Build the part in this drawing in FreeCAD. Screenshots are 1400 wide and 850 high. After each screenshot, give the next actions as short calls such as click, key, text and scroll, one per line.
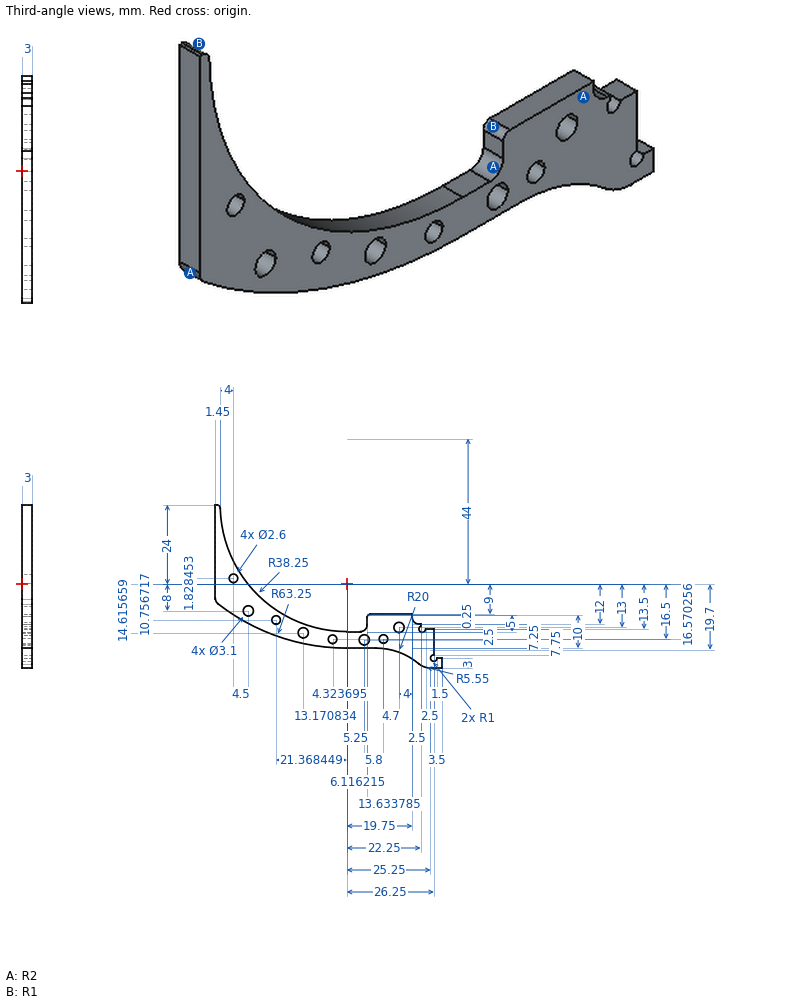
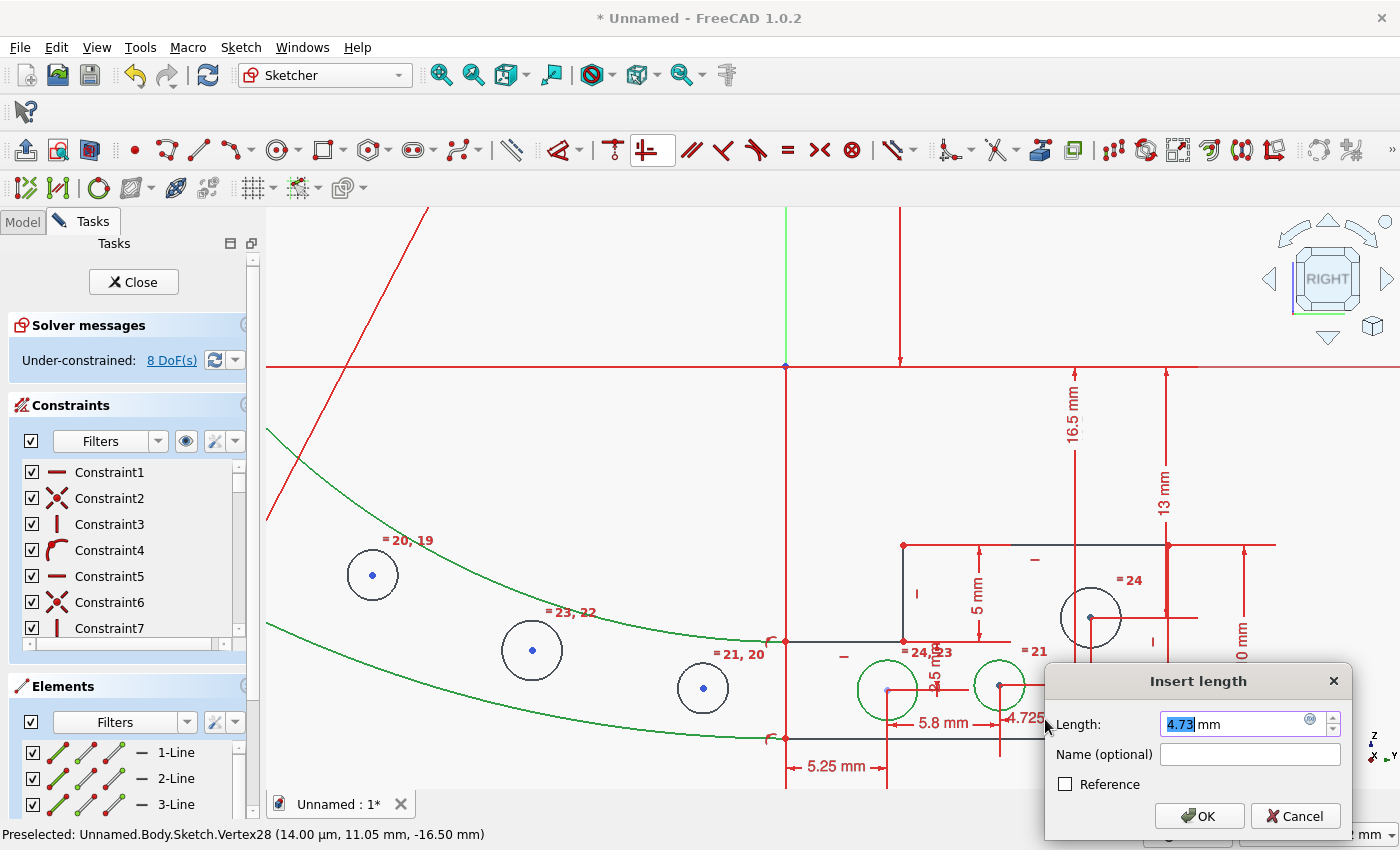
text(4.7)
key(Return)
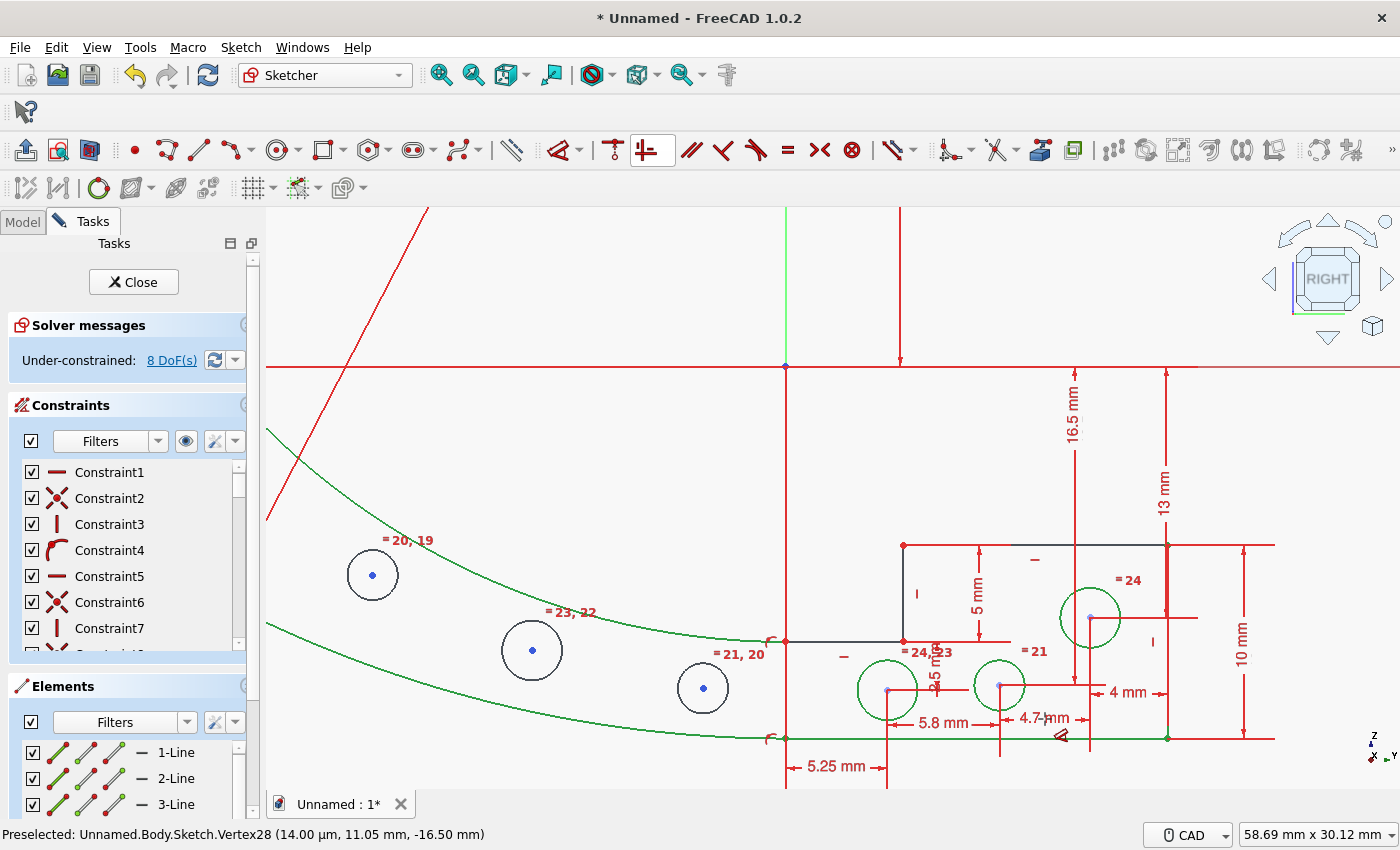
click(868, 642)
click(845, 676)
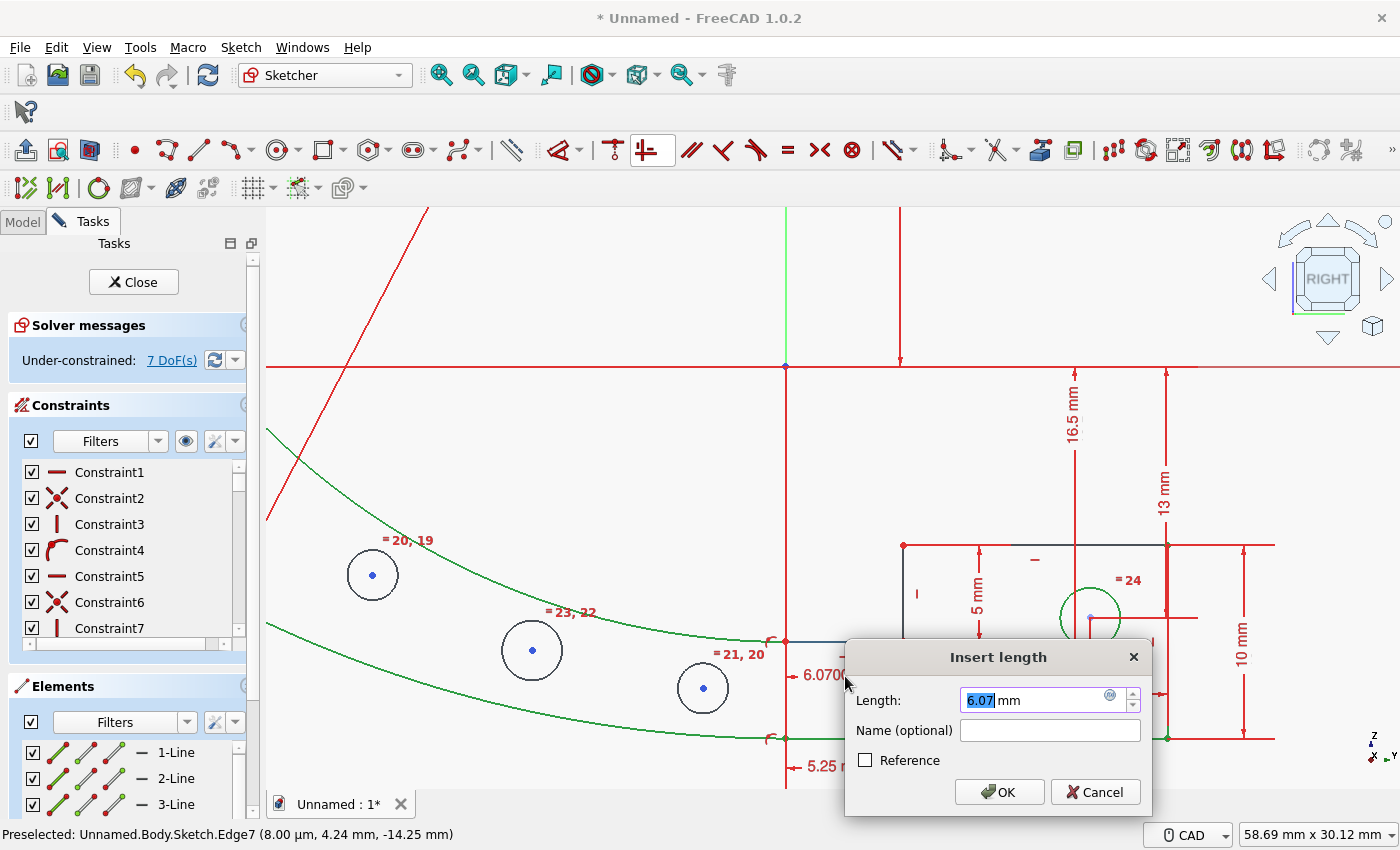
text(6.116215)
key(Return)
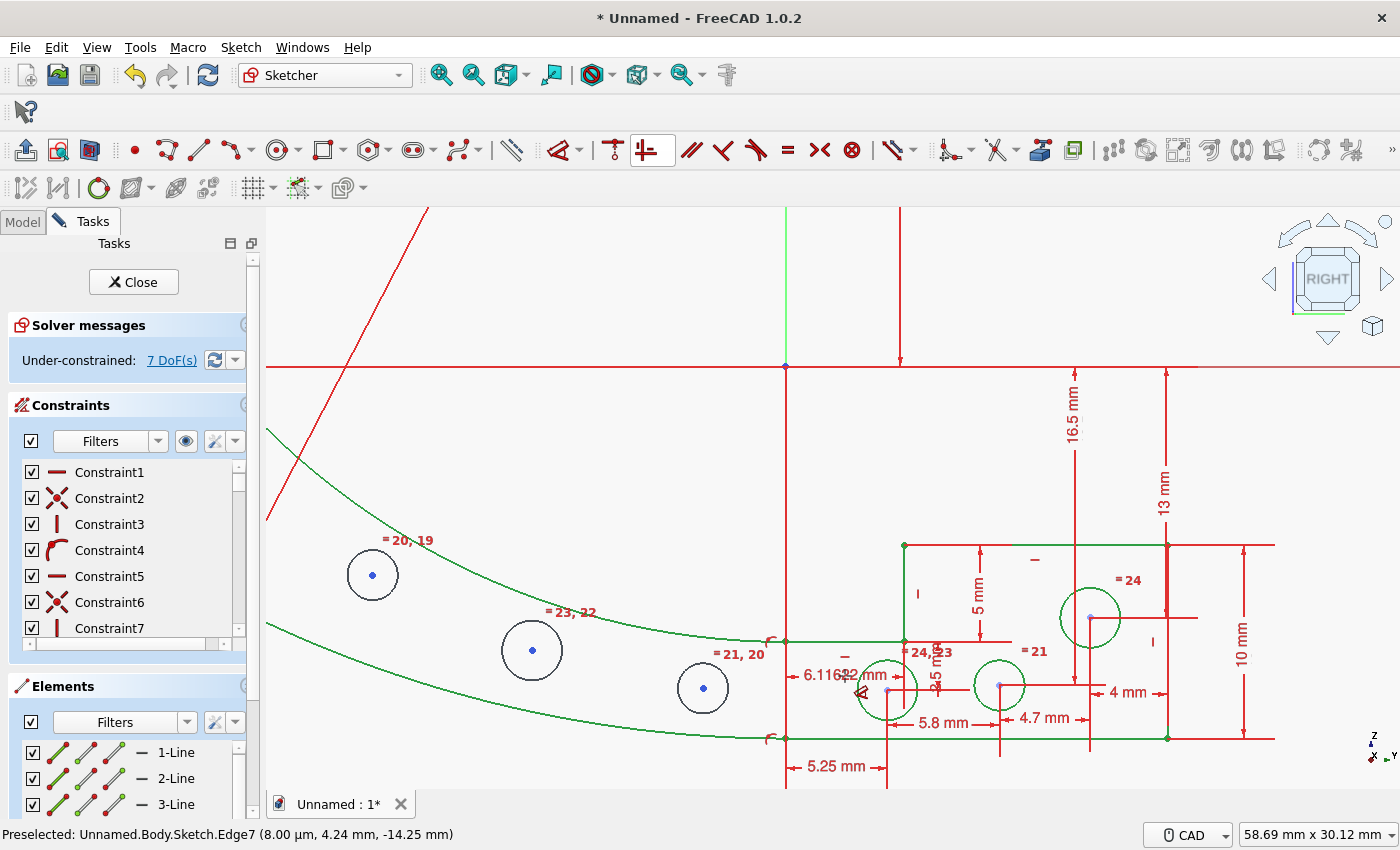
scroll(904, 643, down, 4)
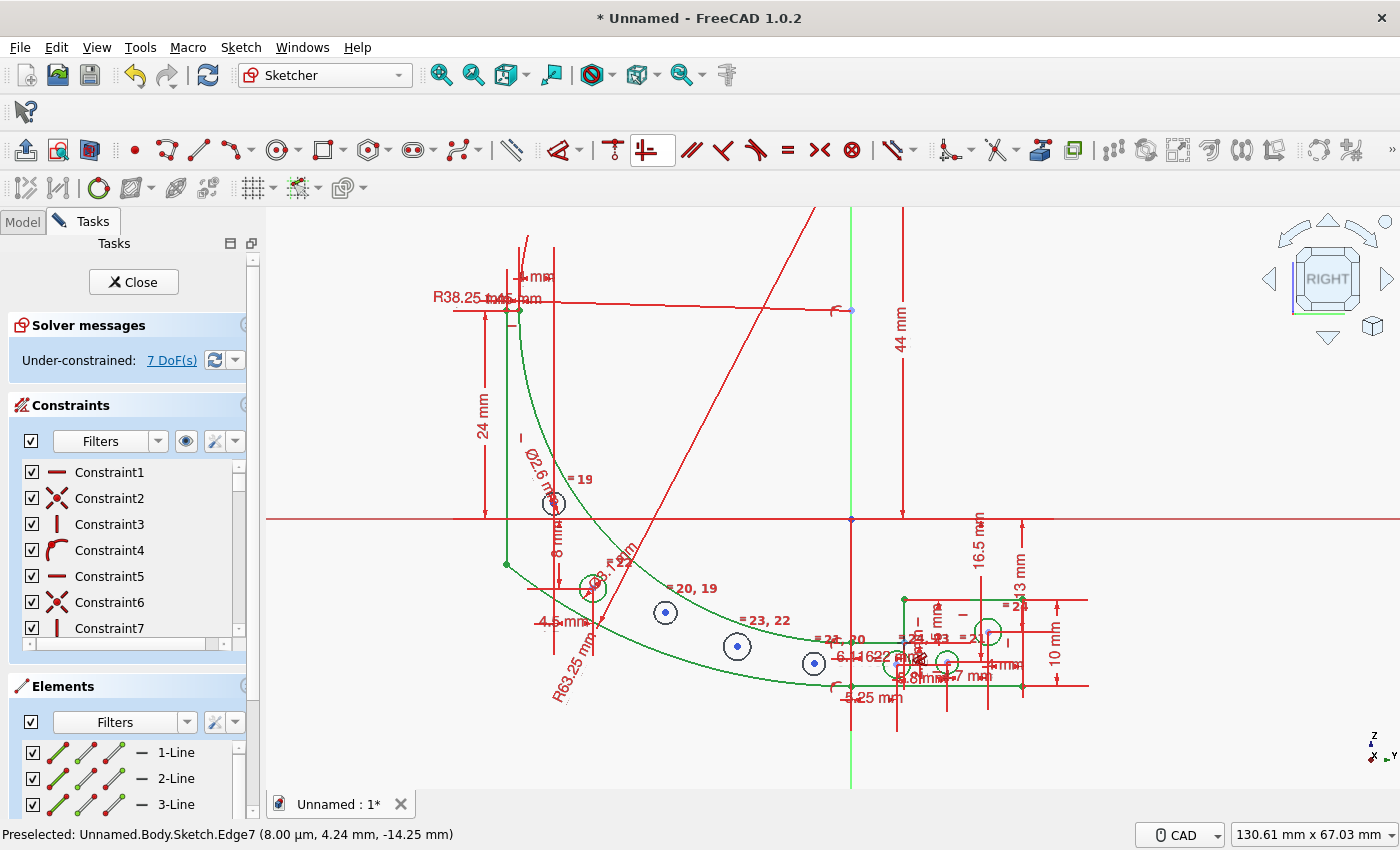
scroll(554, 504, up, 5)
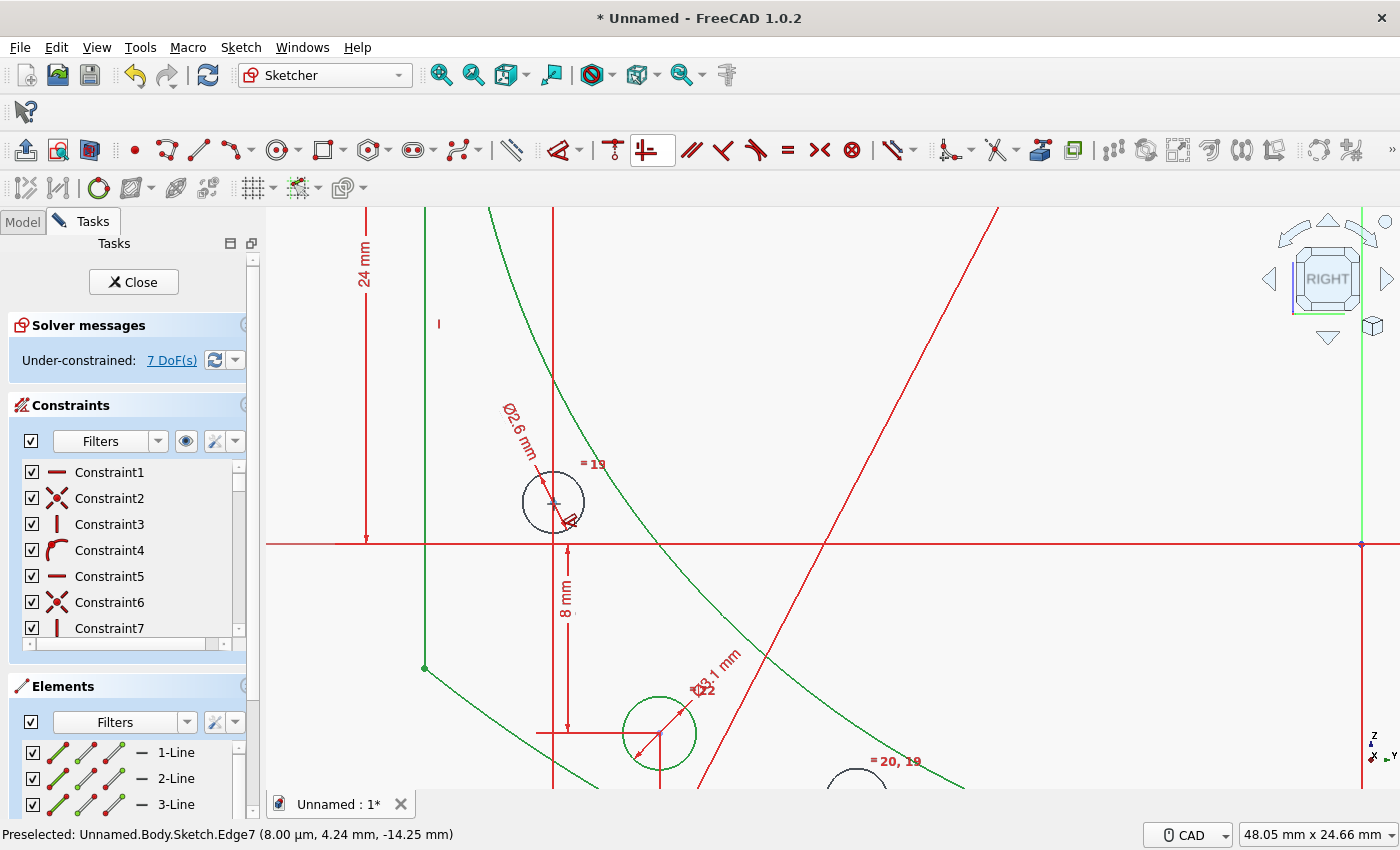
click(553, 502)
click(495, 523)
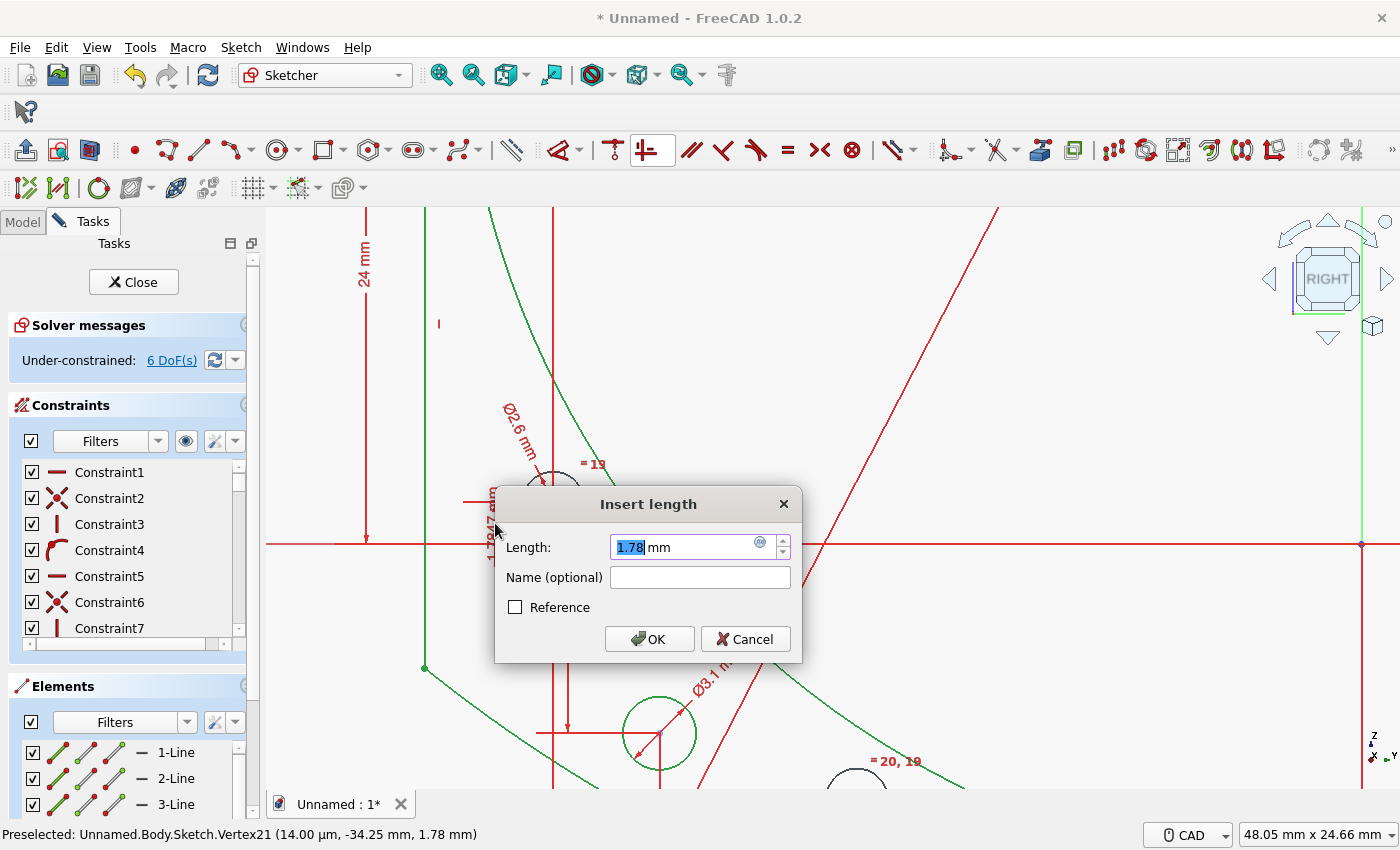
text(1.828453)
key(Return)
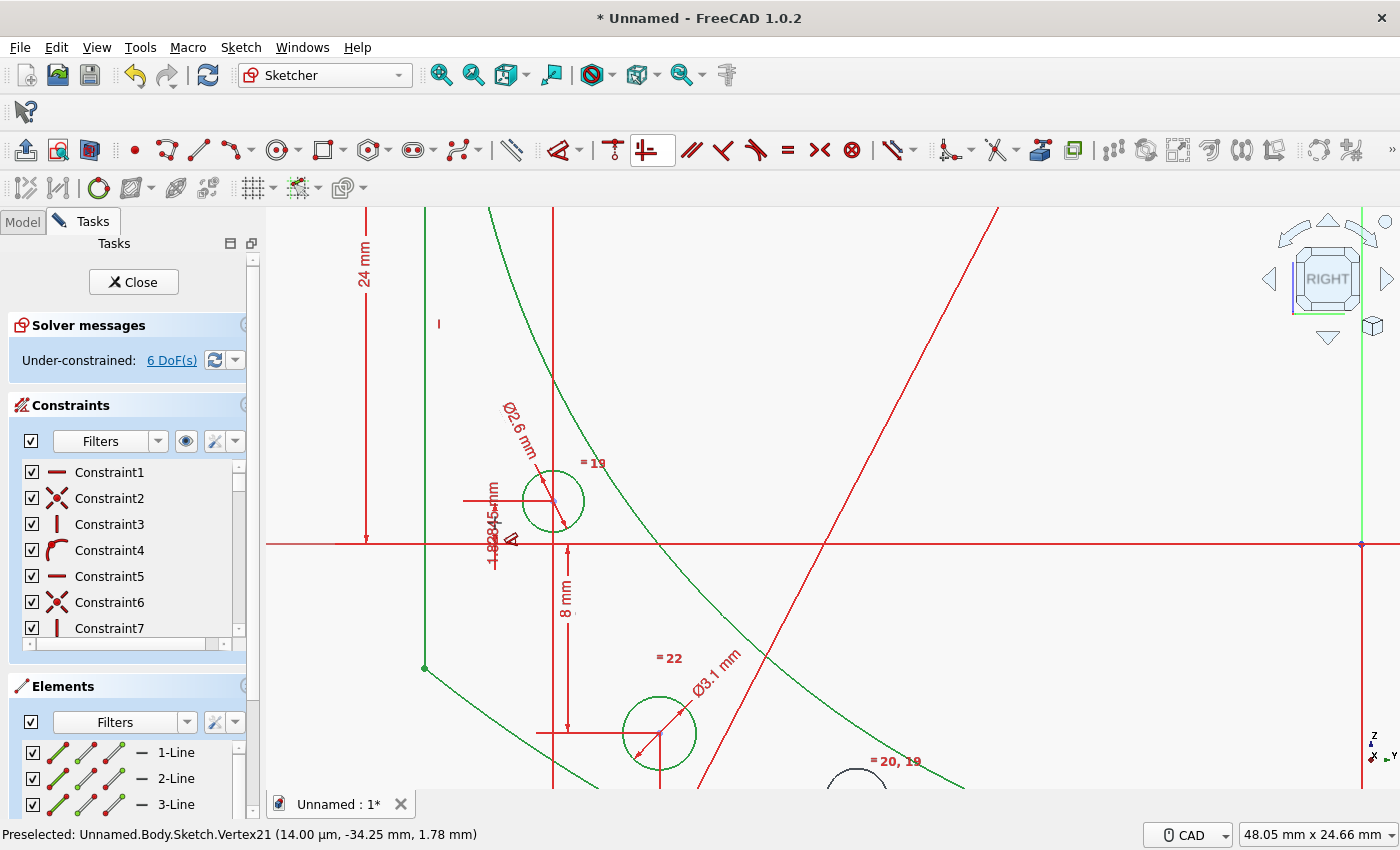
scroll(554, 504, down, 5)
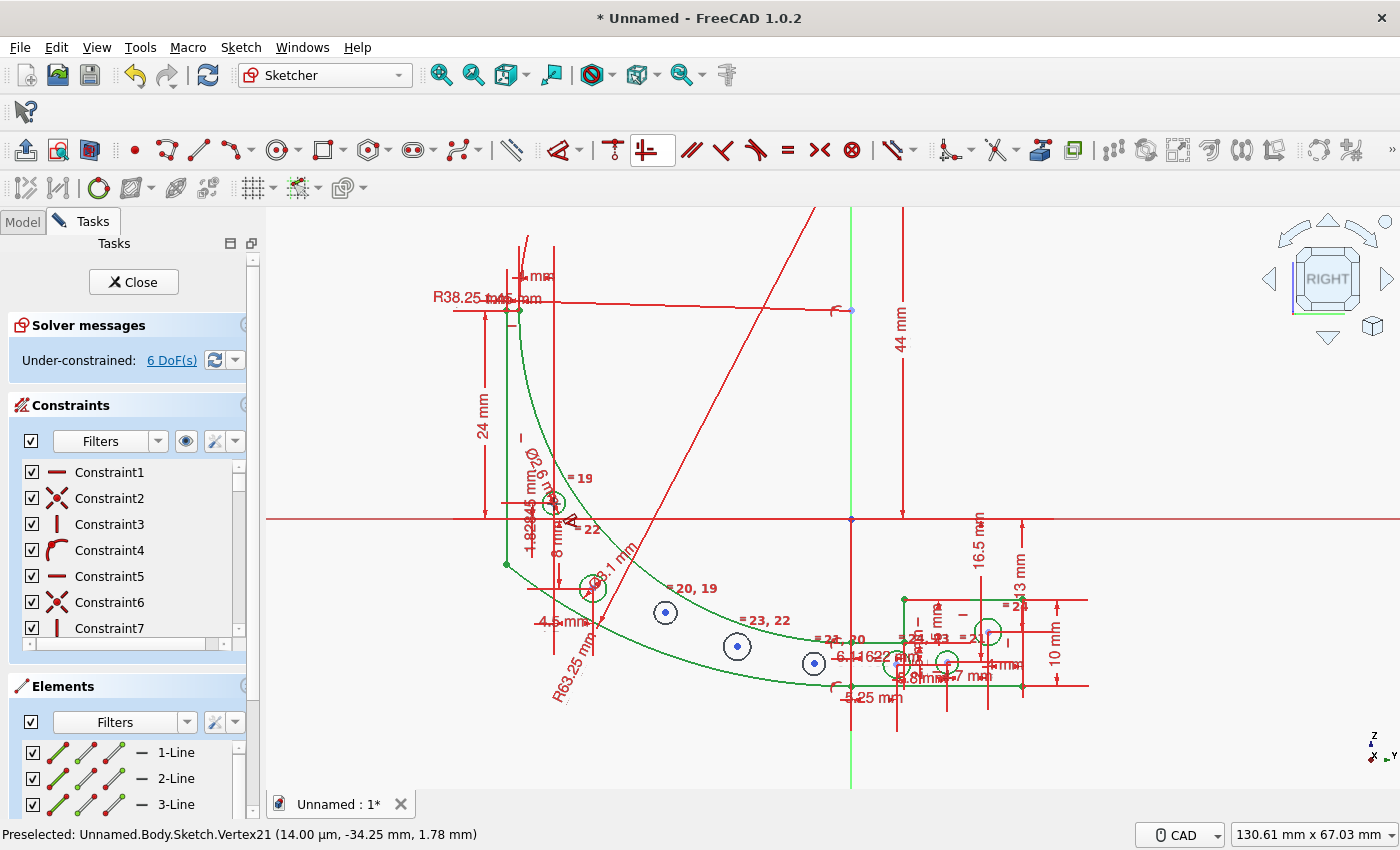
click(814, 664)
click(833, 485)